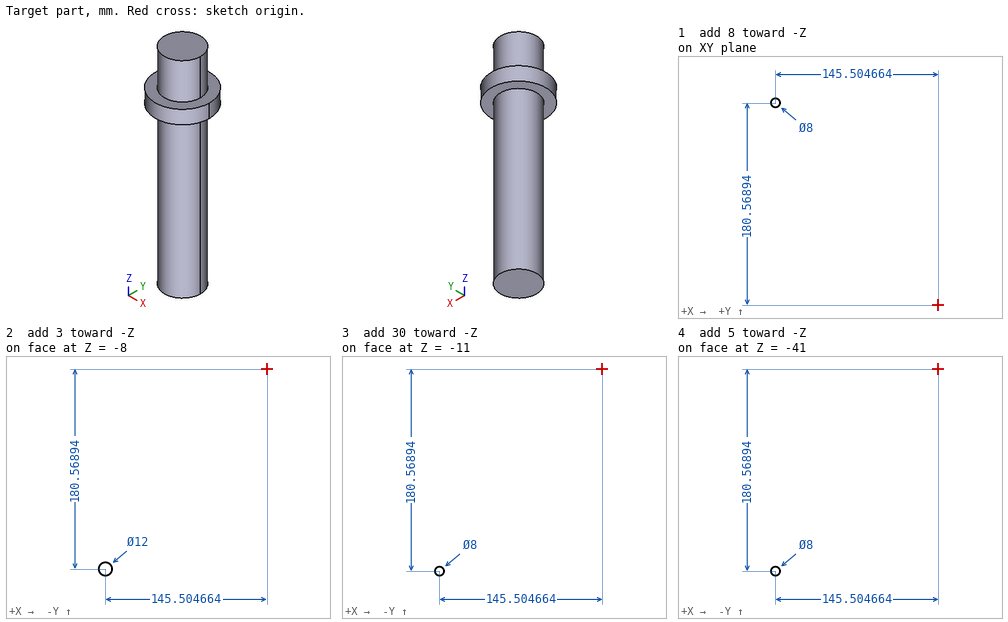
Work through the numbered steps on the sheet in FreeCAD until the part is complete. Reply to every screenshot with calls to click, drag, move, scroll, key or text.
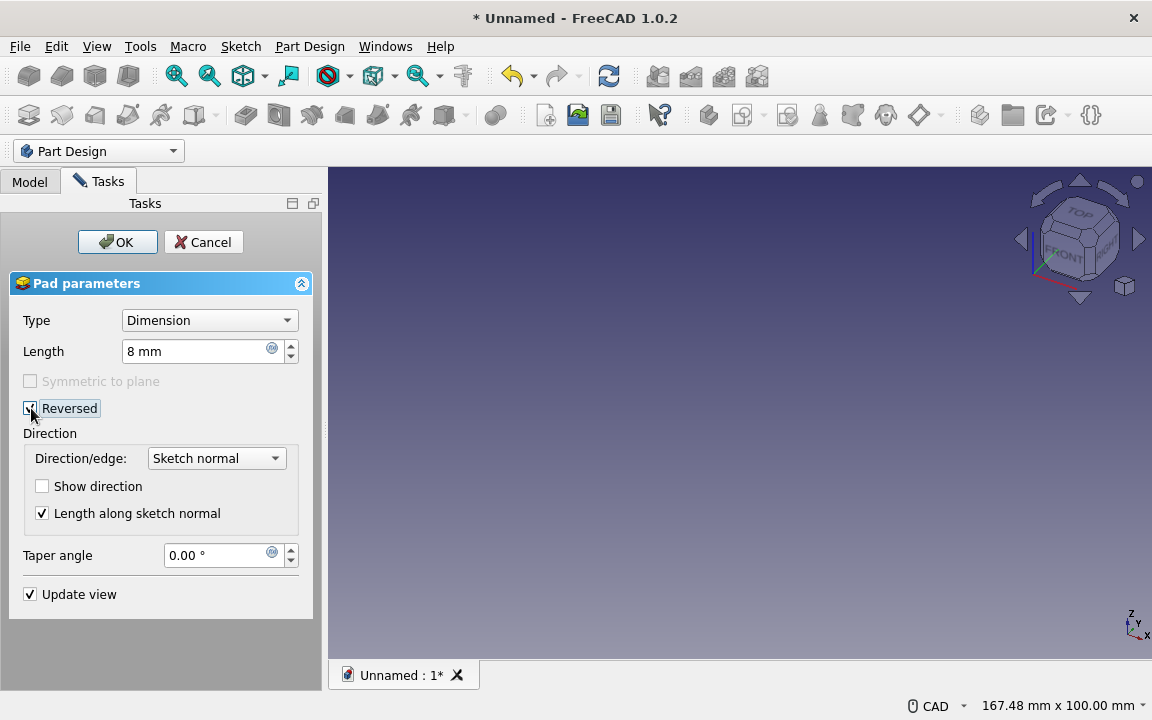
click(118, 242)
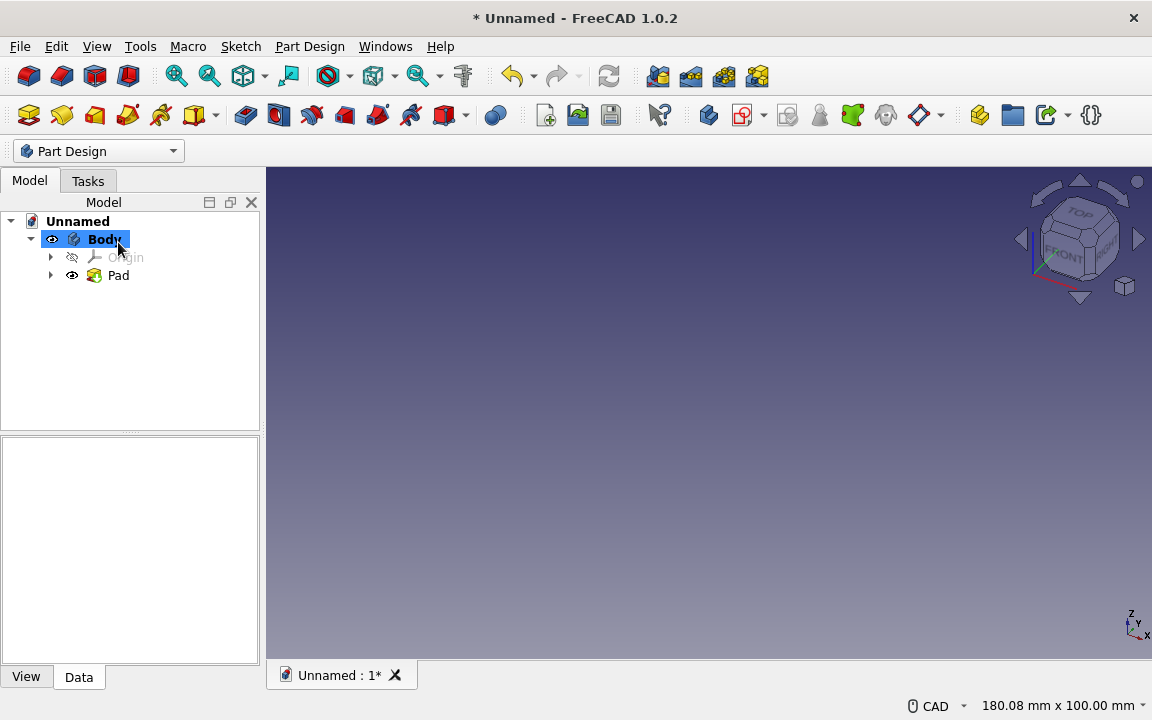
key(v)
key(f)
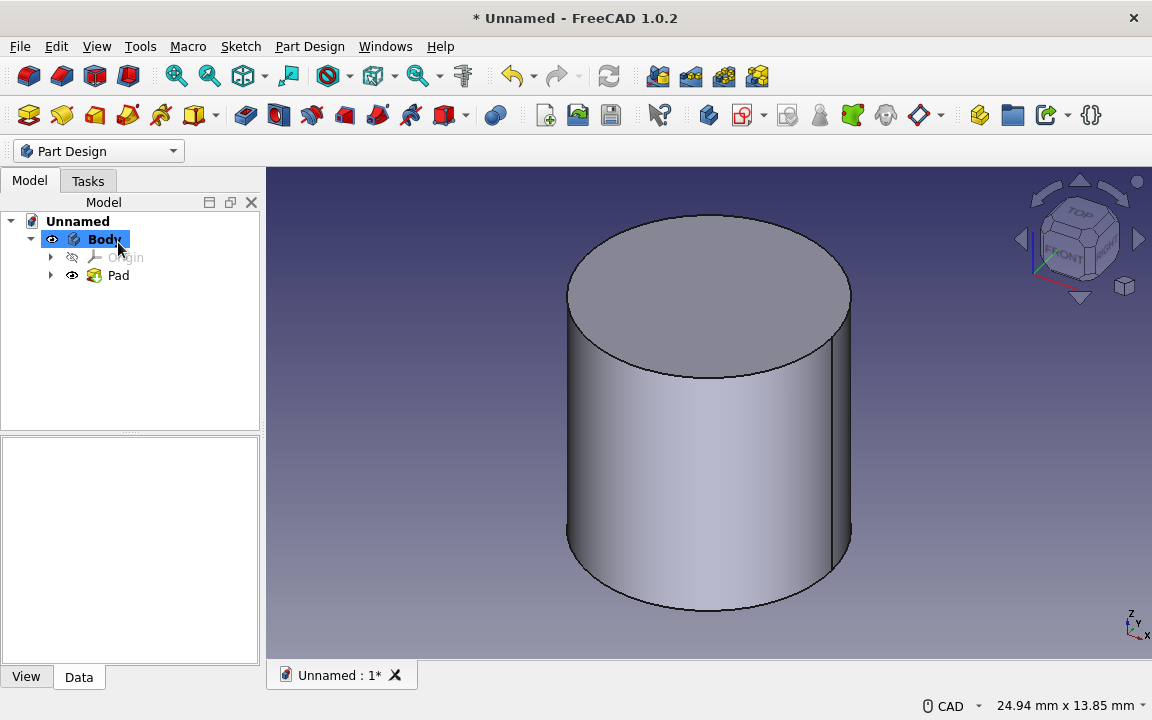
key(5)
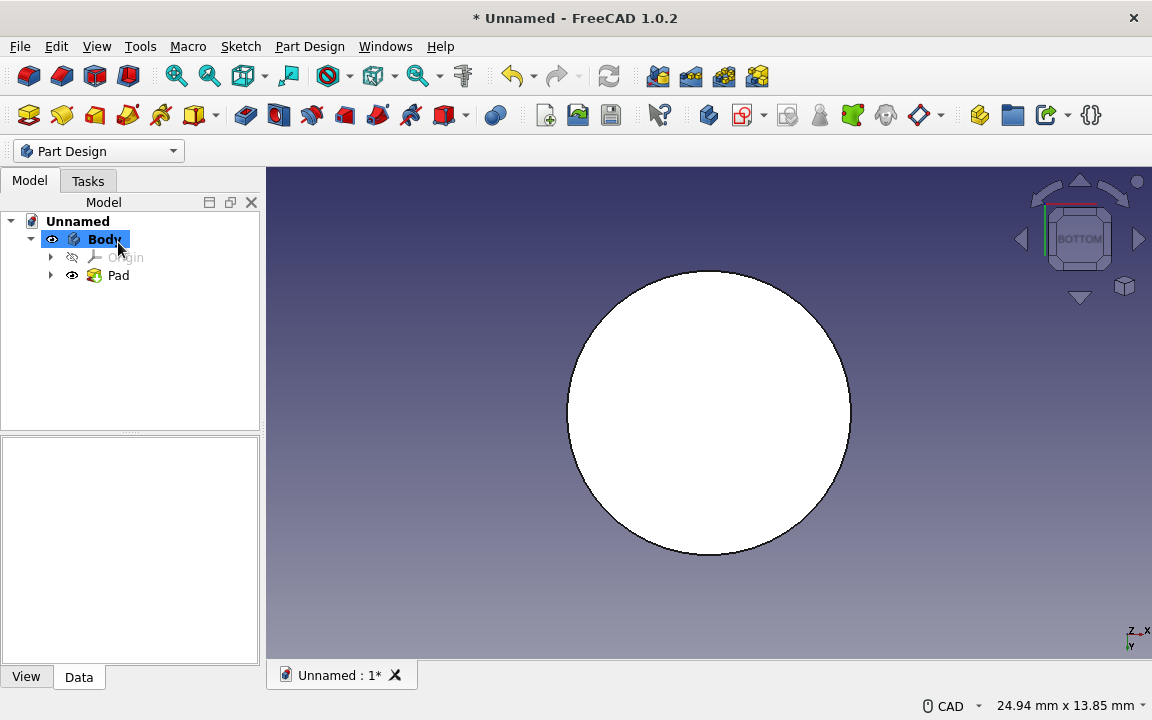
click(709, 412)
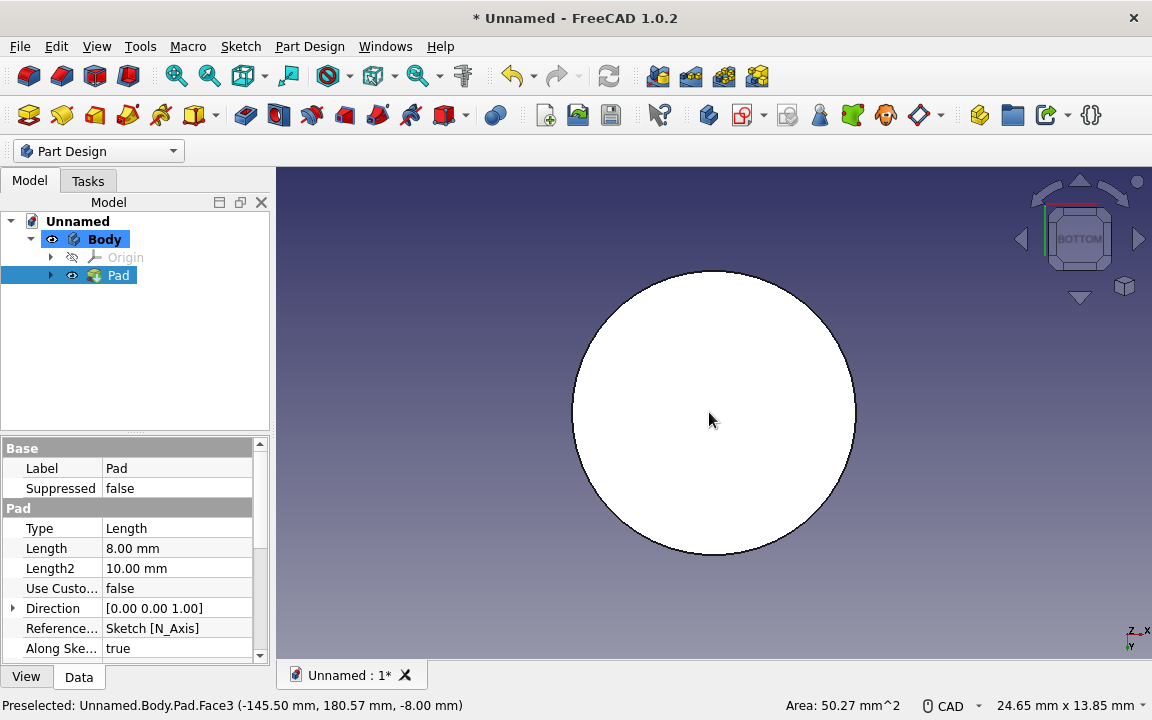
click(742, 116)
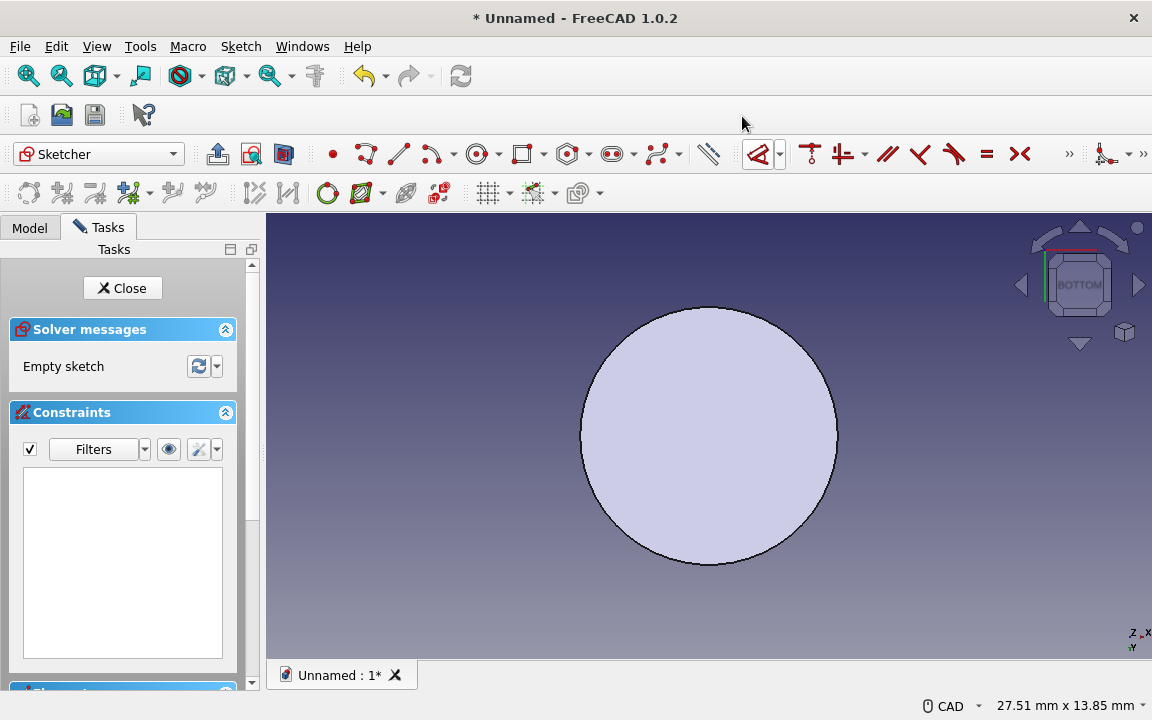
scroll(501, 436, down, 2)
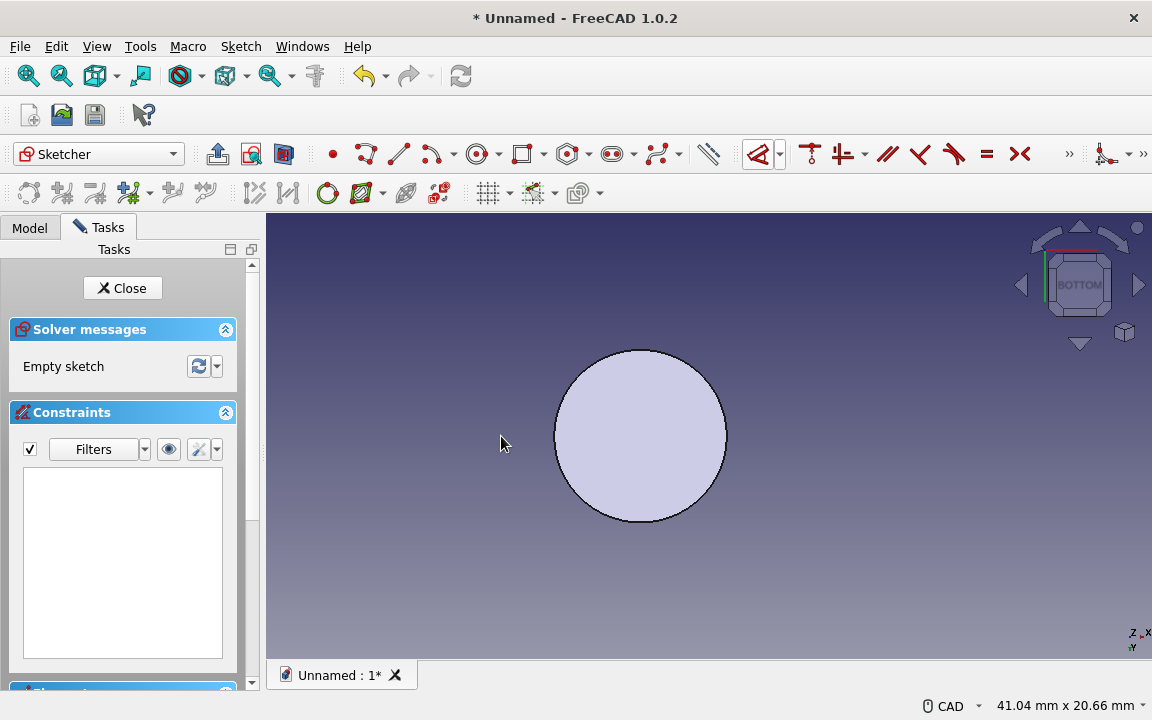
click(476, 154)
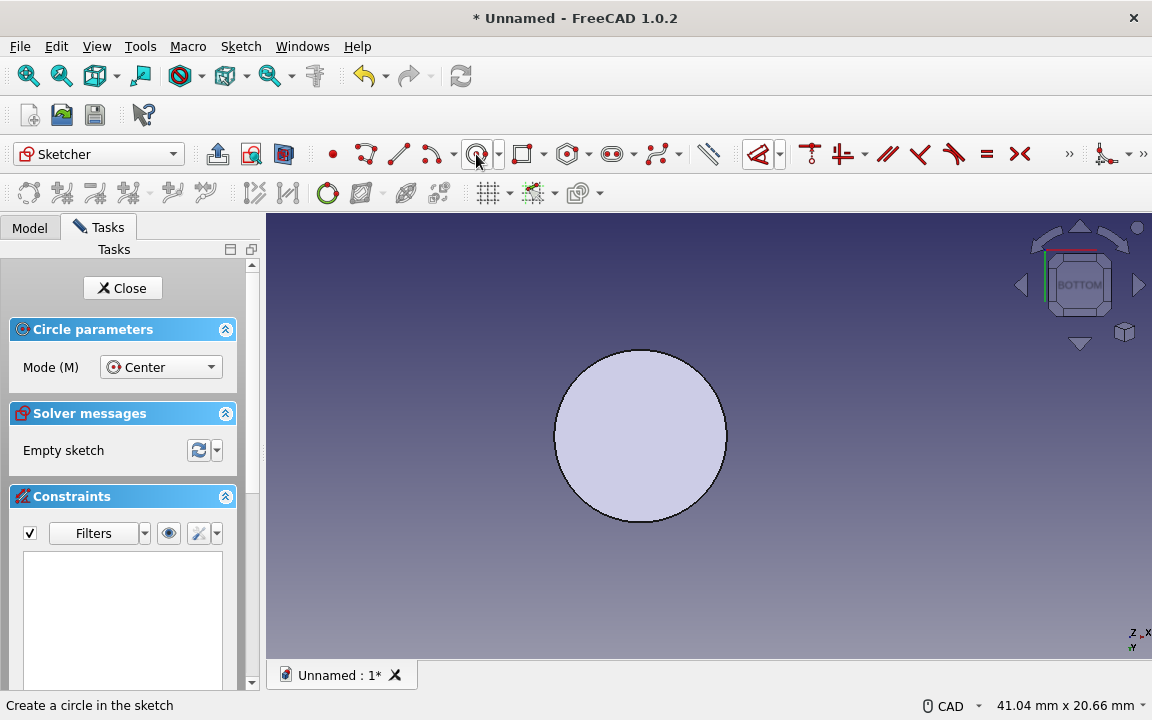
click(641, 436)
click(732, 345)
key(Escape)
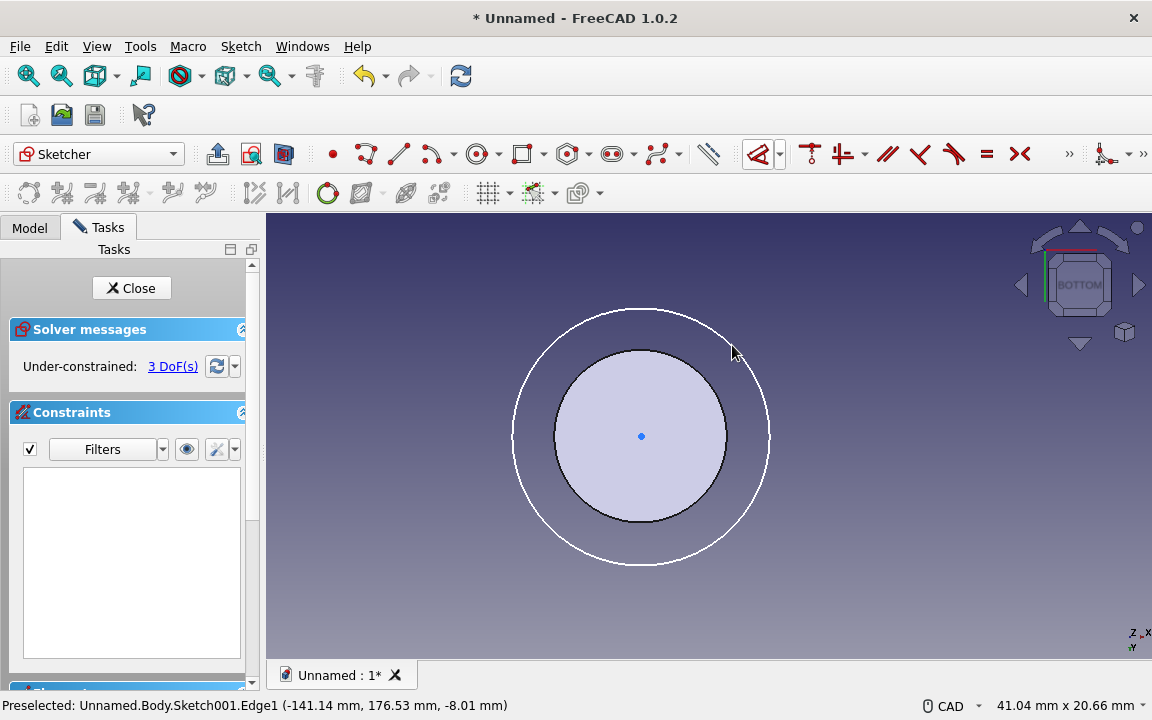
click(732, 346)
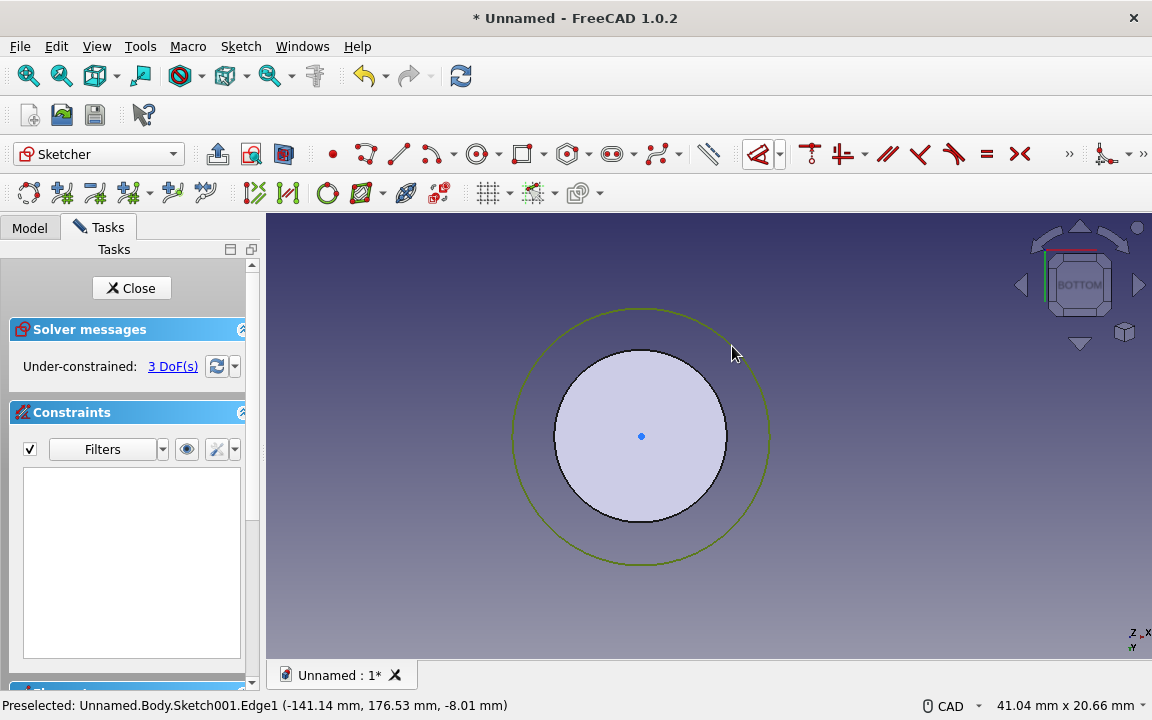
key(k)
key(o)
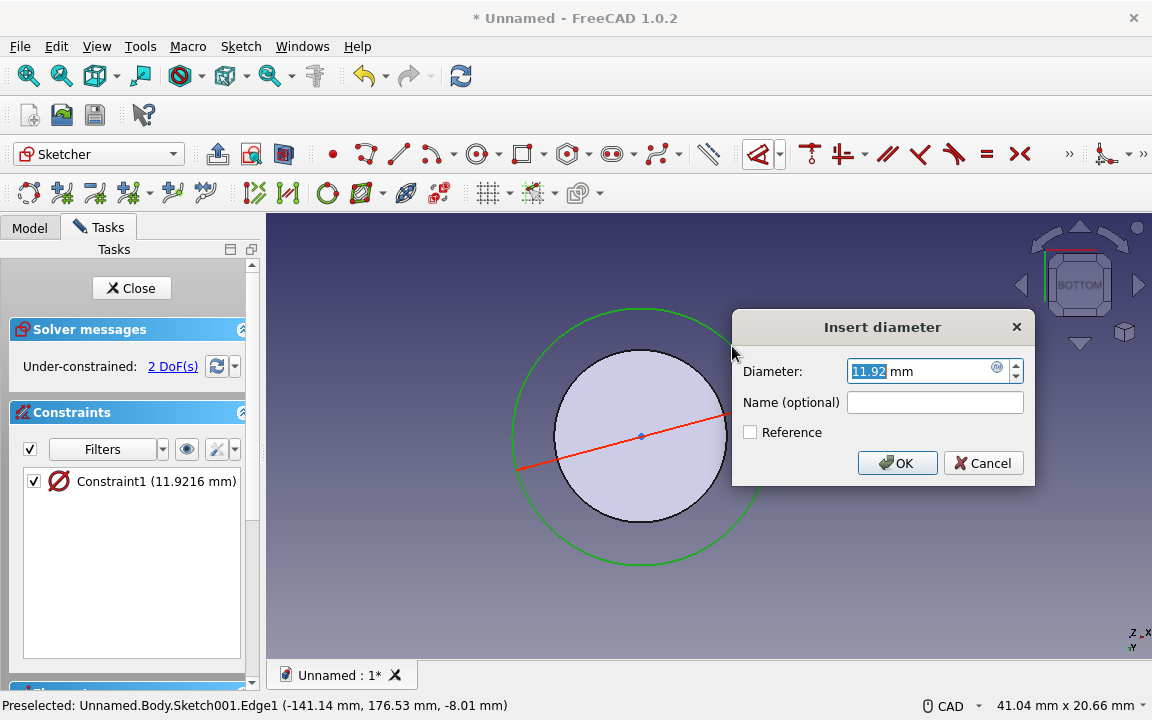
text(12)
key(Return)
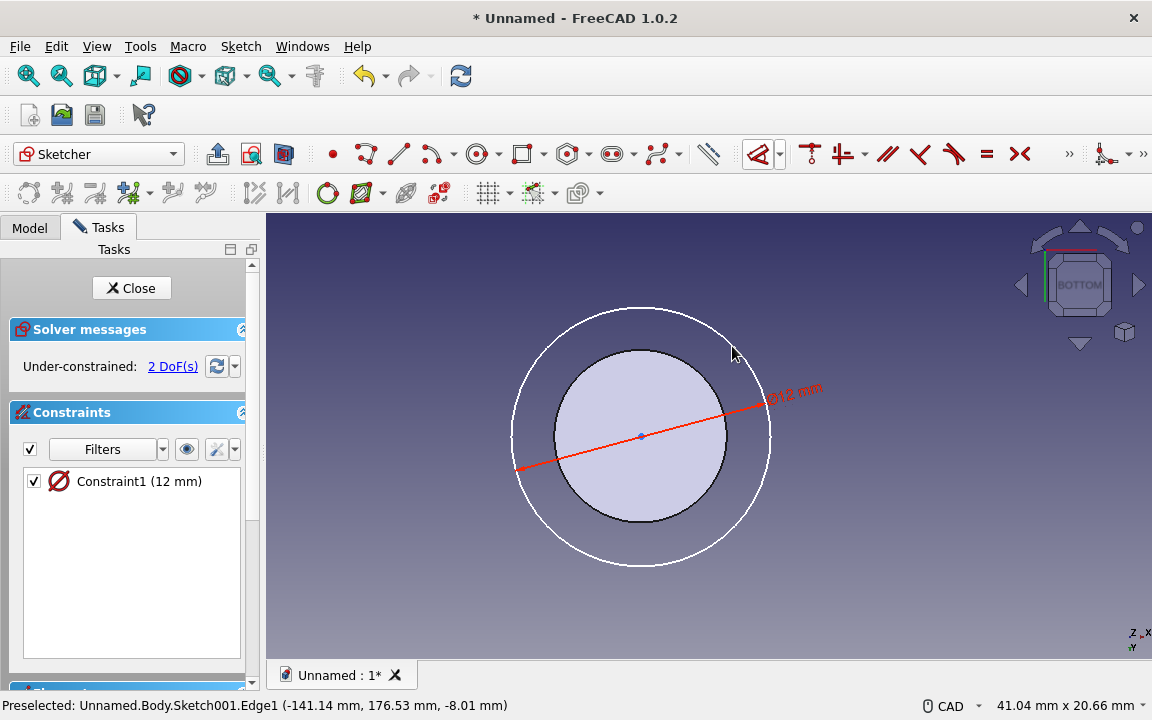
click(641, 437)